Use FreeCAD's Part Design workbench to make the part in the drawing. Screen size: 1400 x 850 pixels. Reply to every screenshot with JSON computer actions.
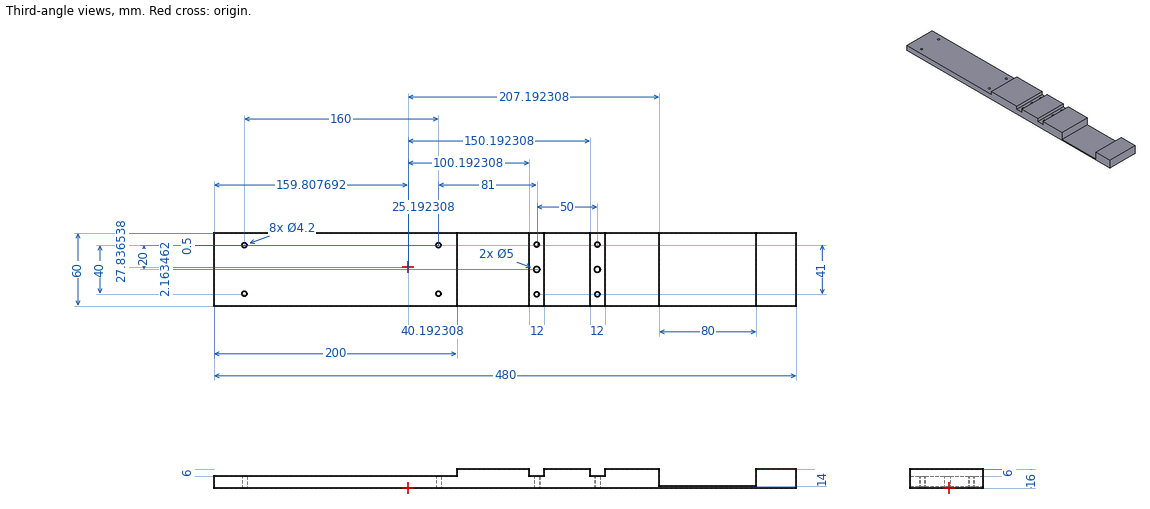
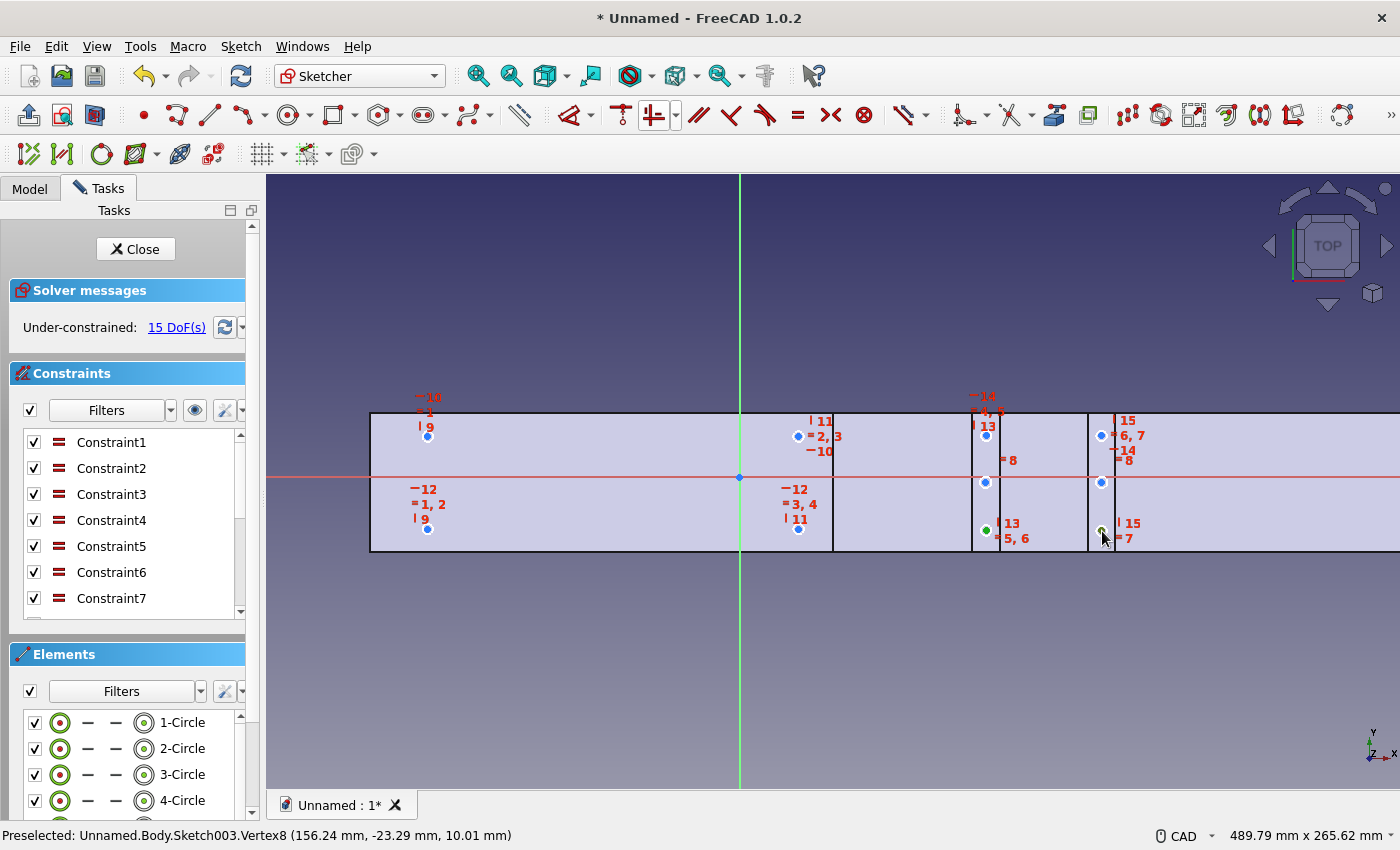
{"action": "left_click", "coordinate": [676, 116]}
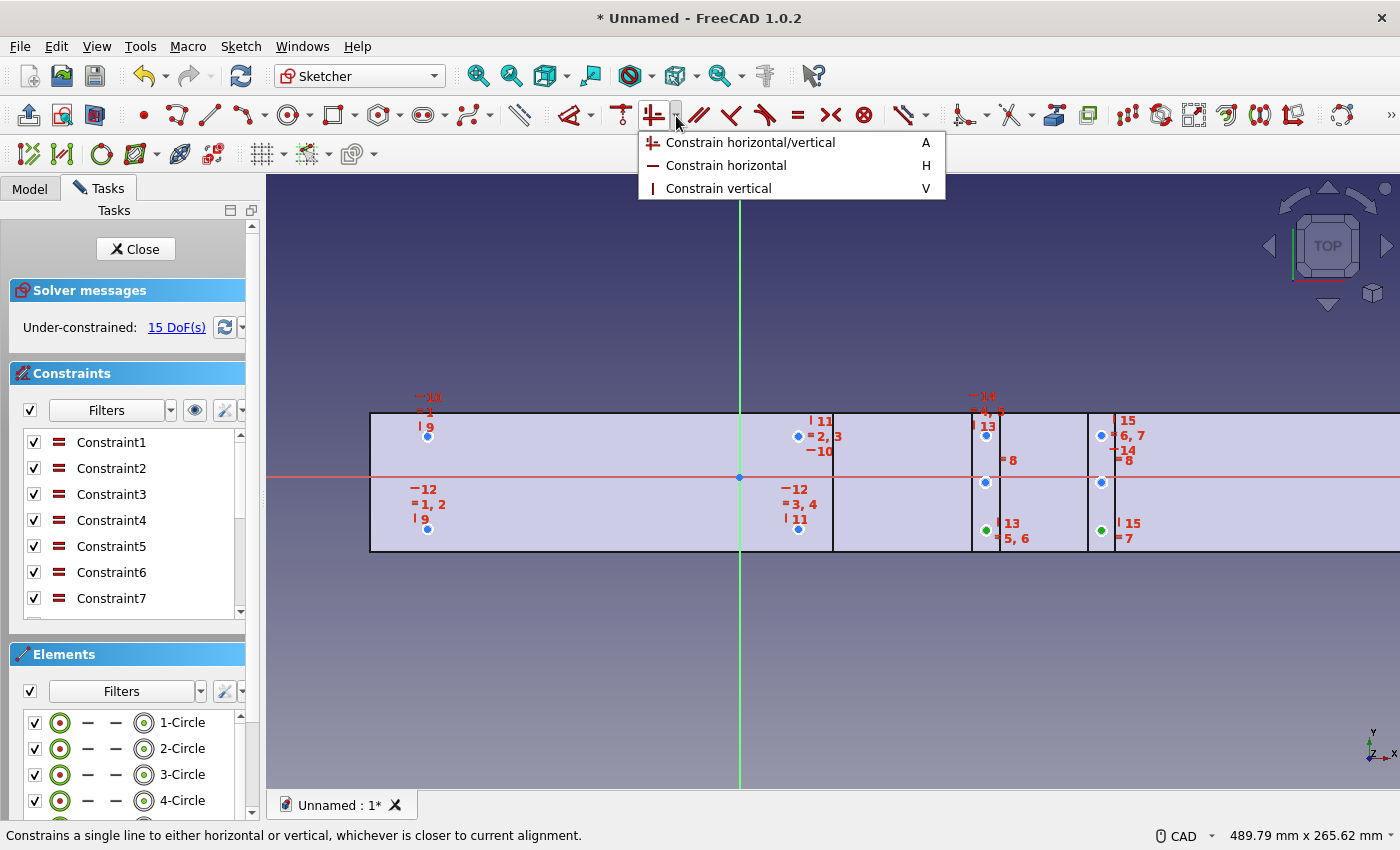
{"action": "left_click", "coordinate": [792, 166]}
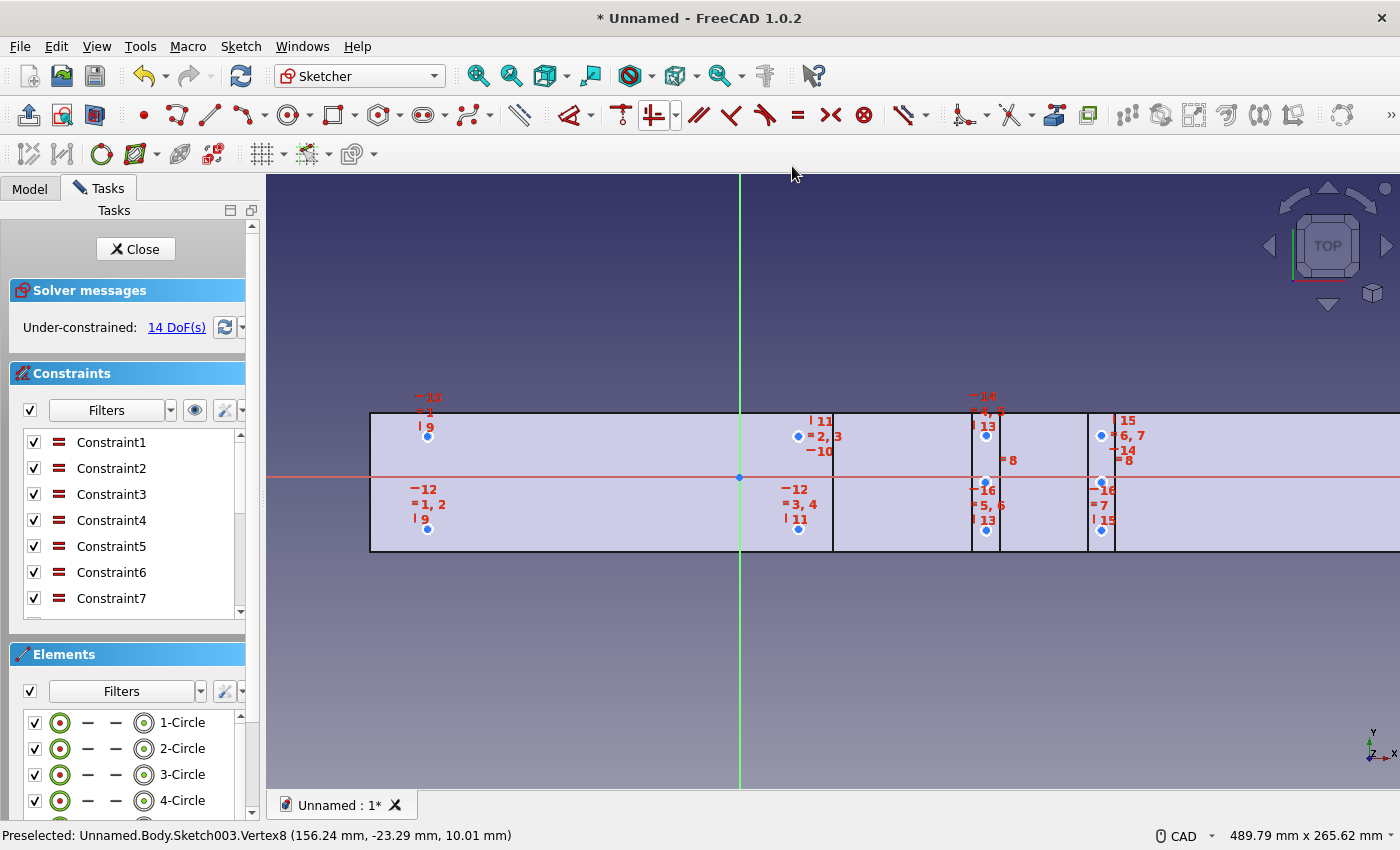
{"action": "left_click", "coordinate": [986, 436]}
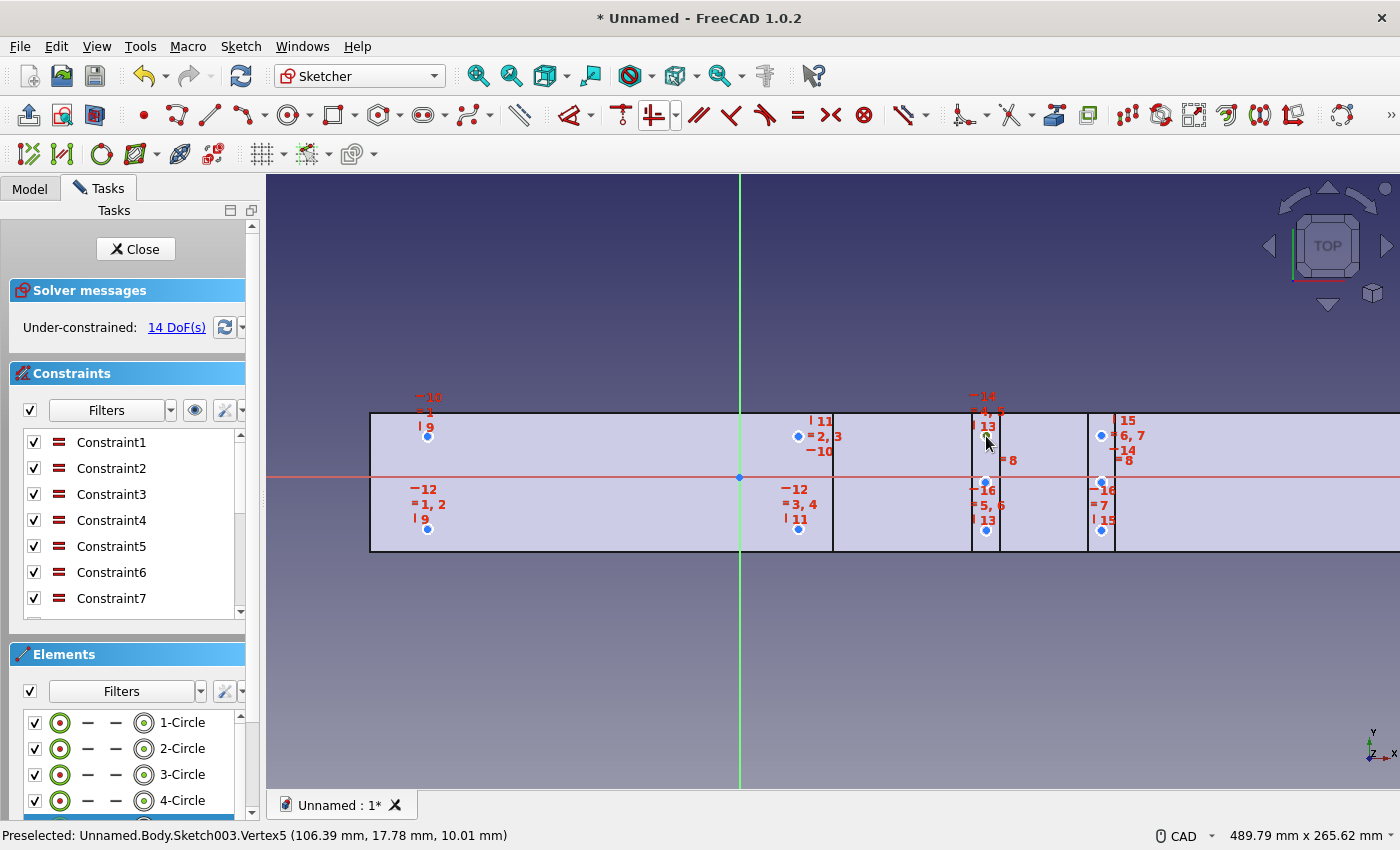
{"action": "left_click", "coordinate": [986, 482]}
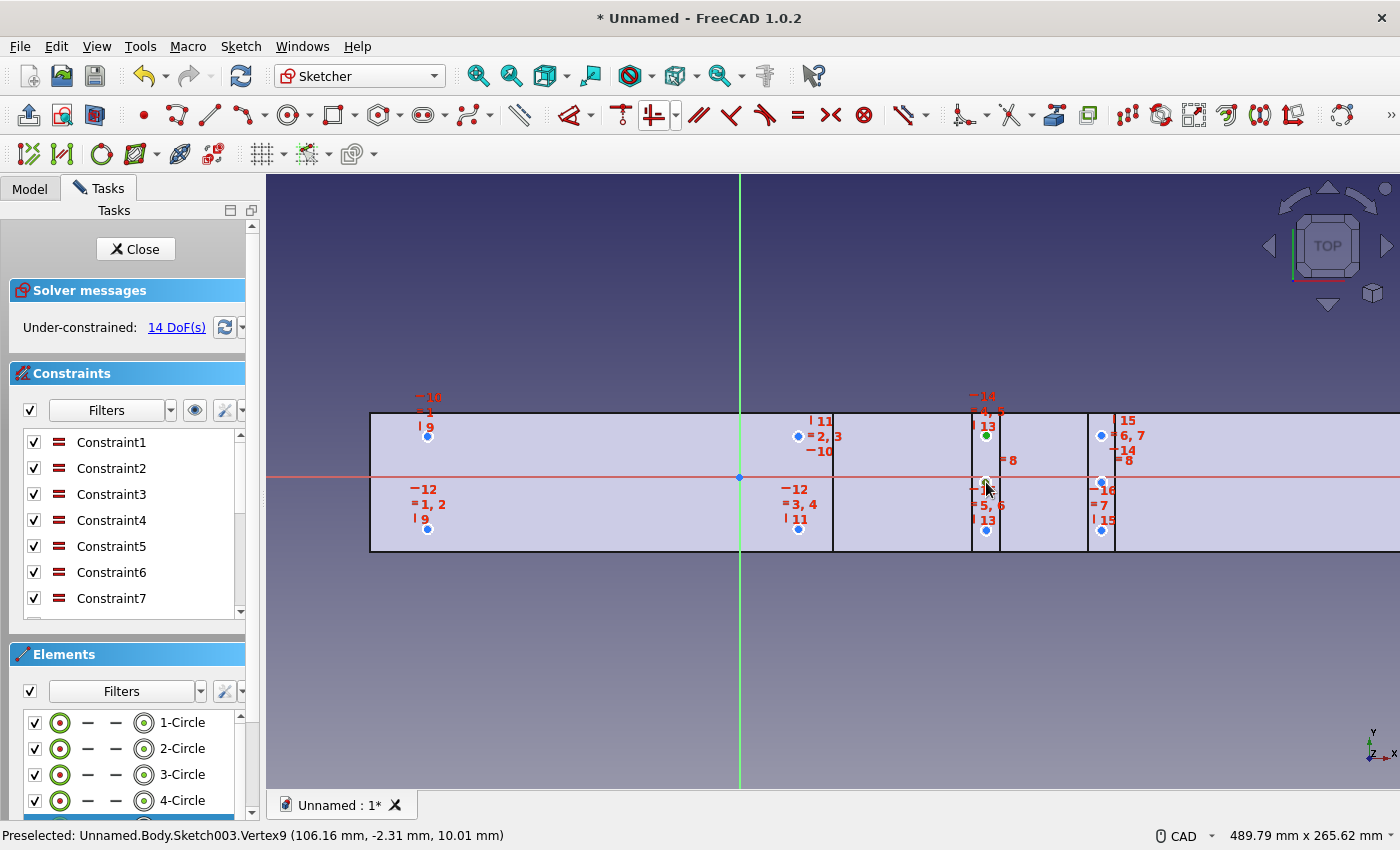
{"action": "key", "text": "v"}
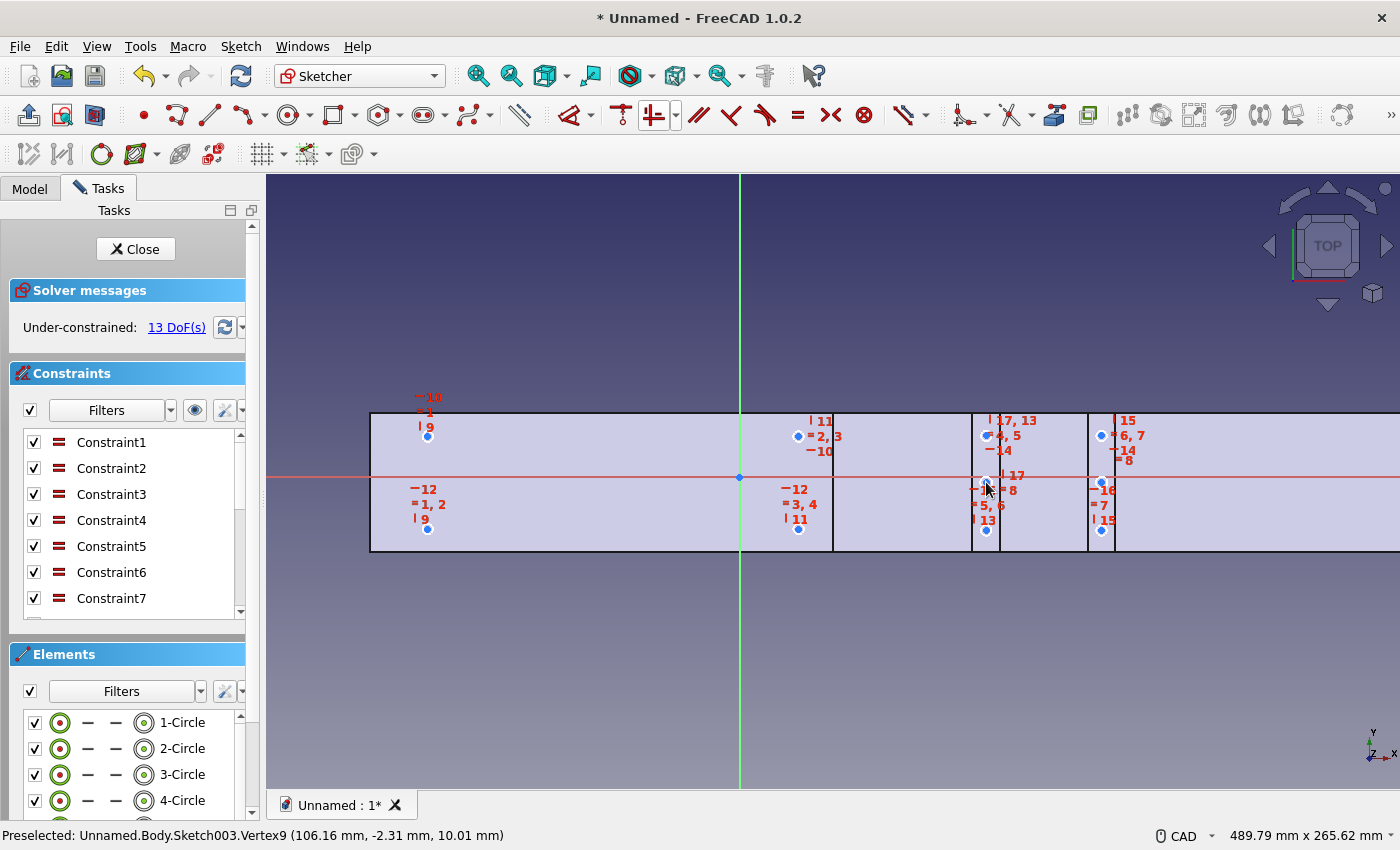
{"action": "left_click", "coordinate": [1102, 436]}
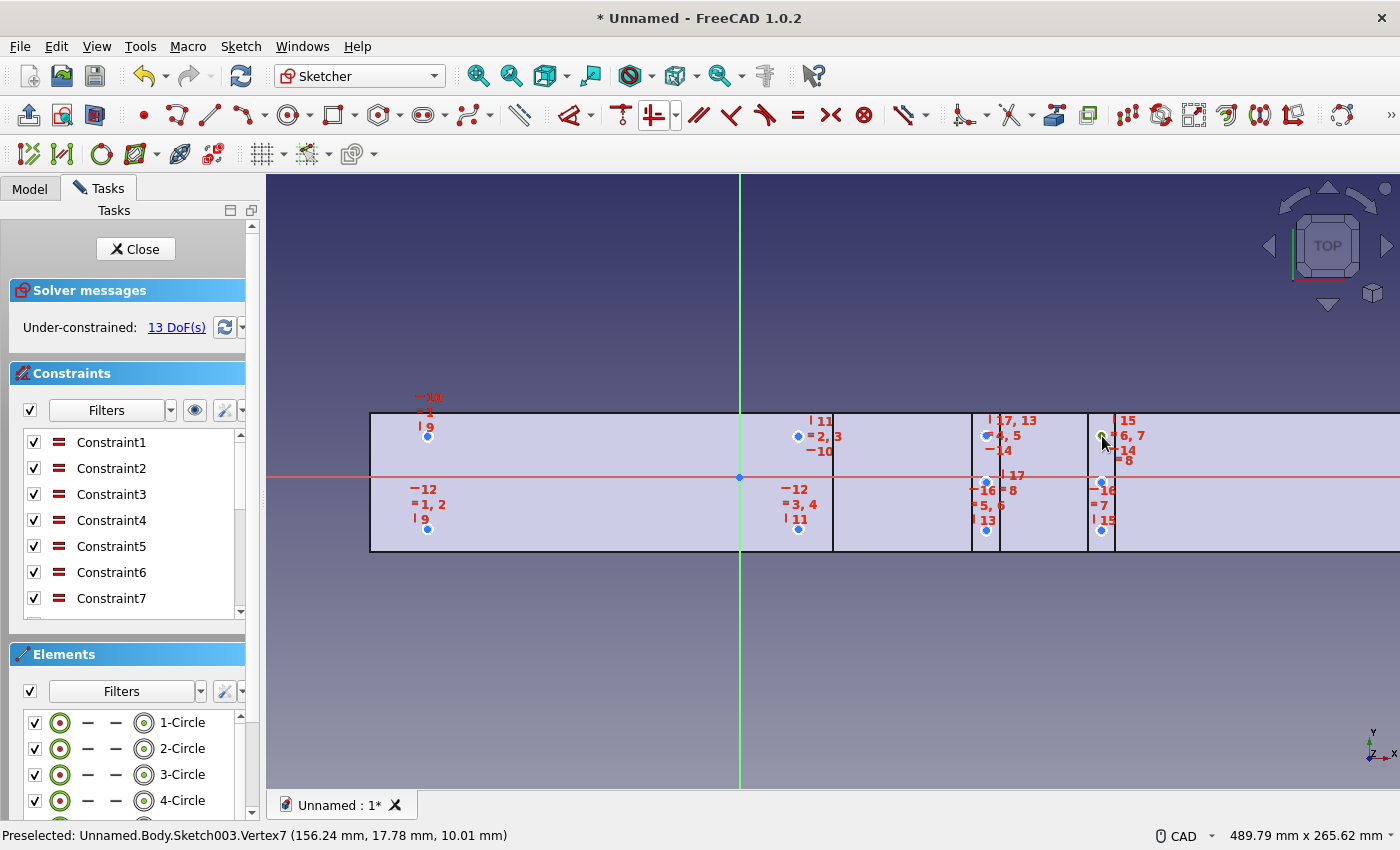
{"action": "left_click", "coordinate": [1102, 482]}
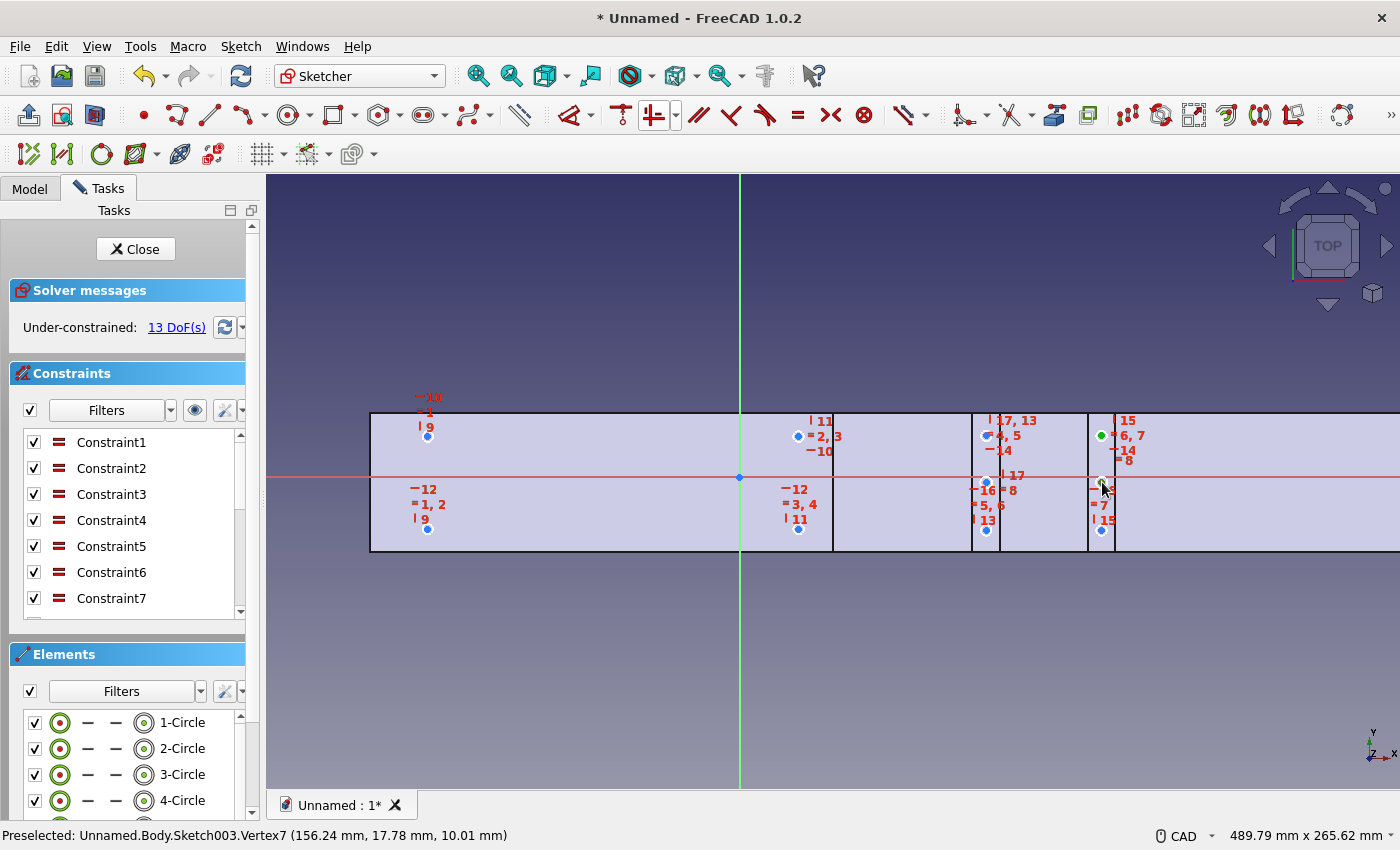
{"action": "key", "text": "v"}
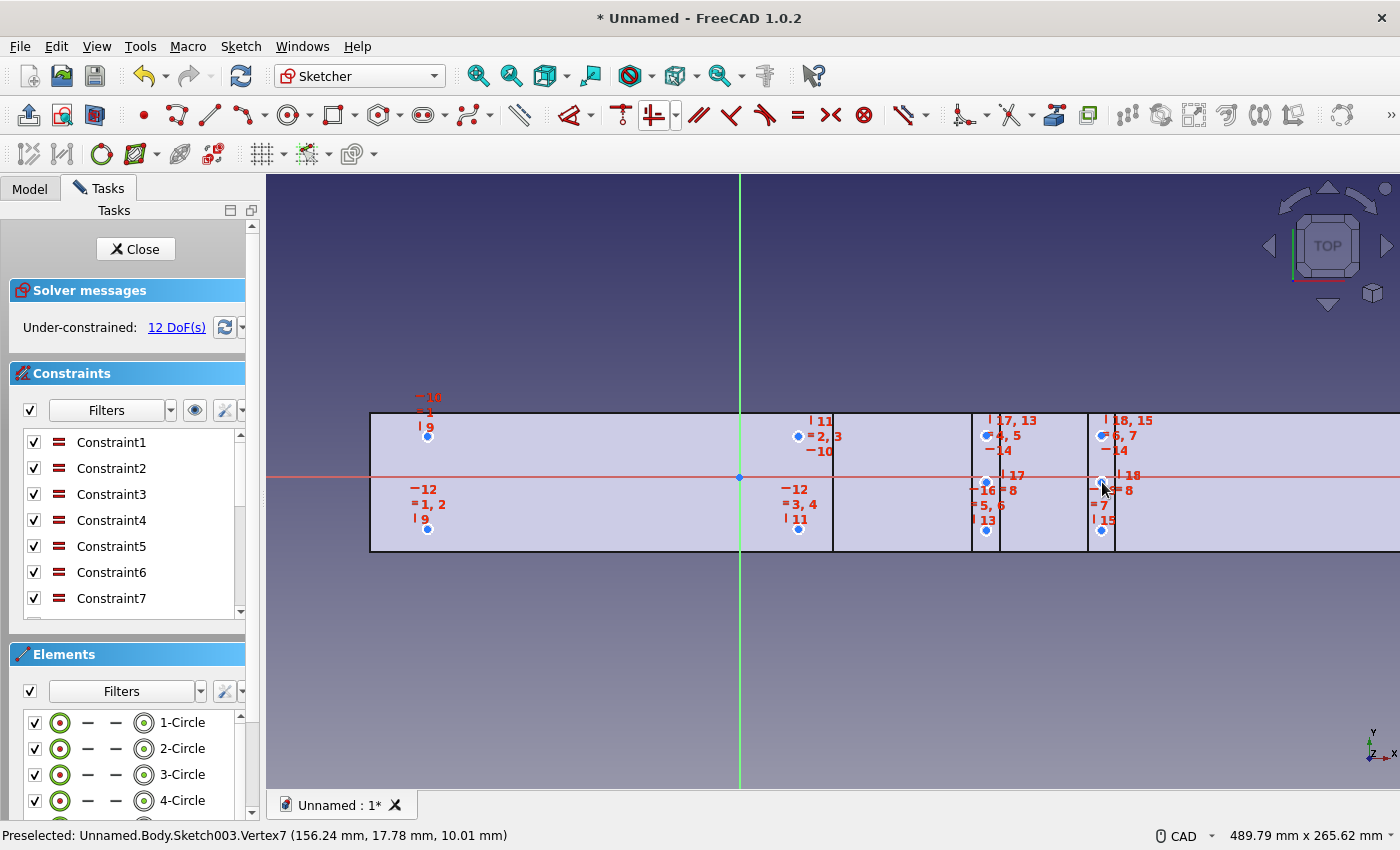
{"action": "left_click", "coordinate": [986, 482]}